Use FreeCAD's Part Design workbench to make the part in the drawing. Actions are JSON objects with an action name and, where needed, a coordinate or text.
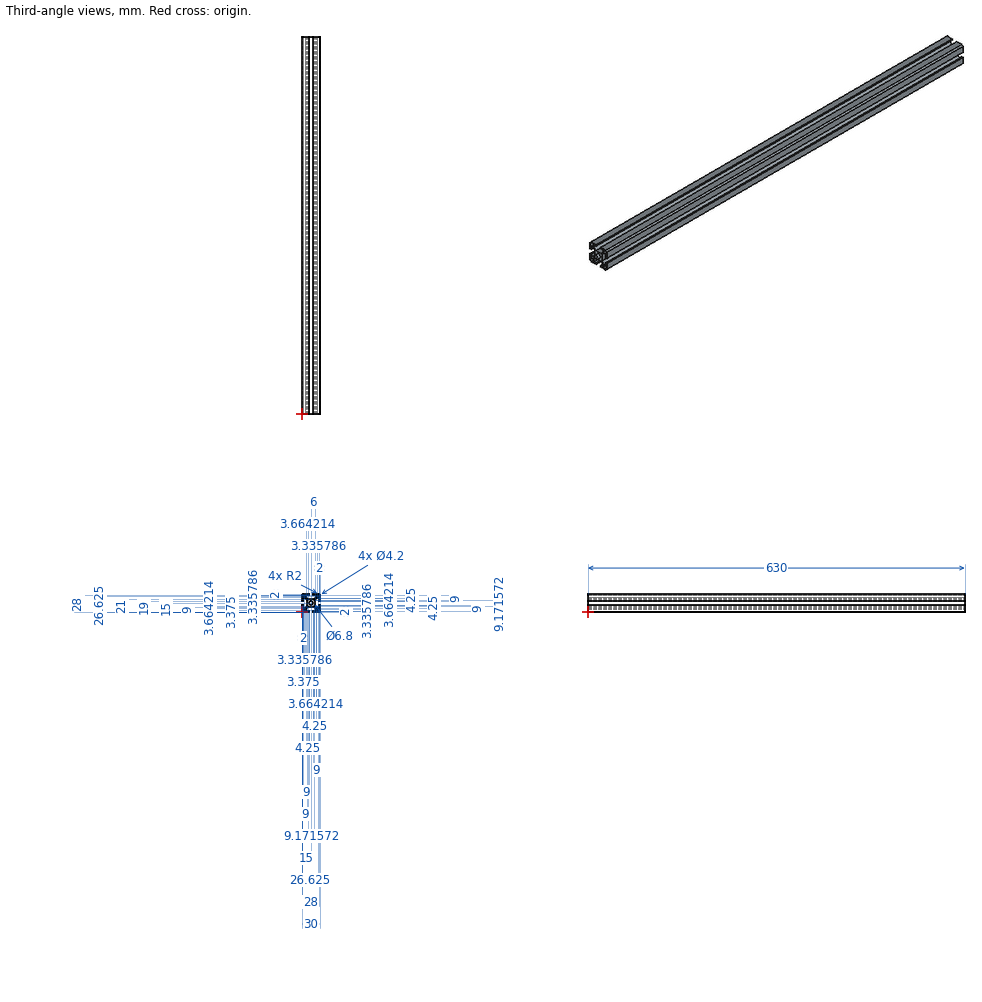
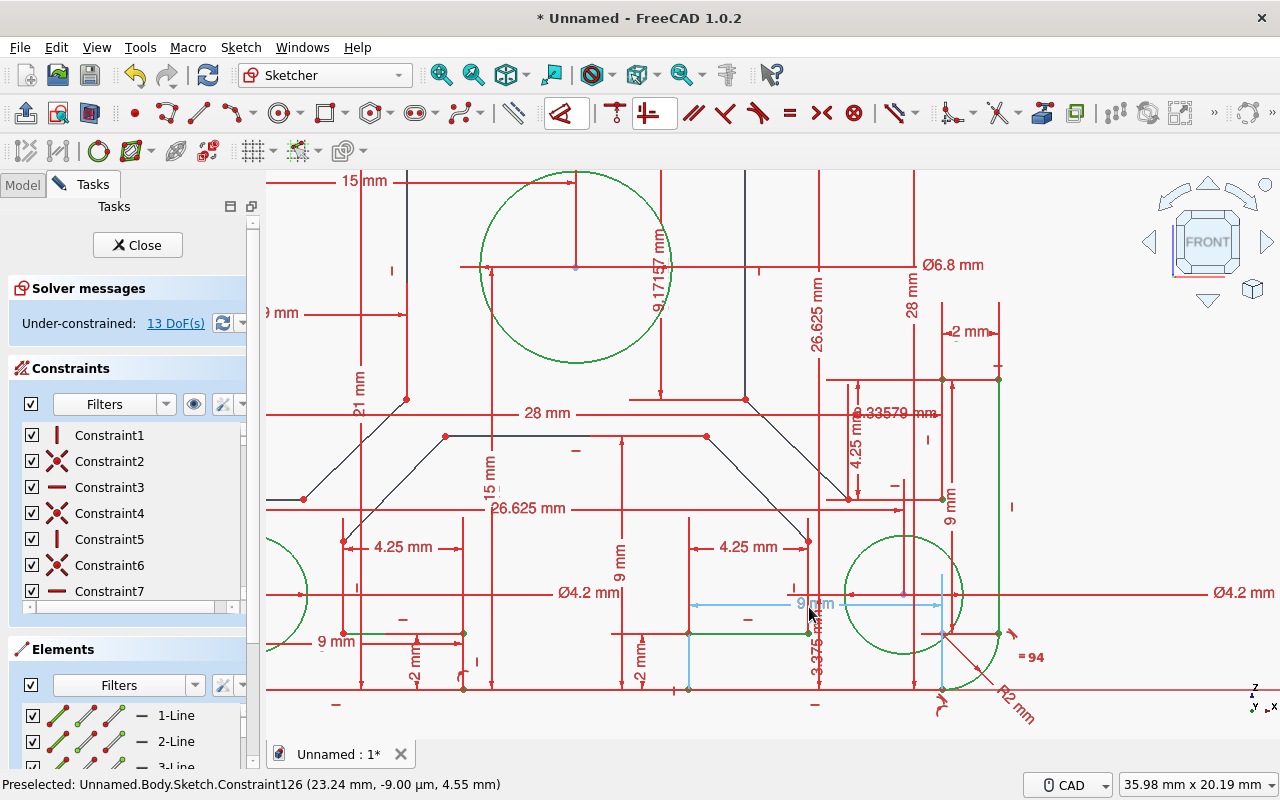
{"action": "left_click", "coordinate": [808, 569]}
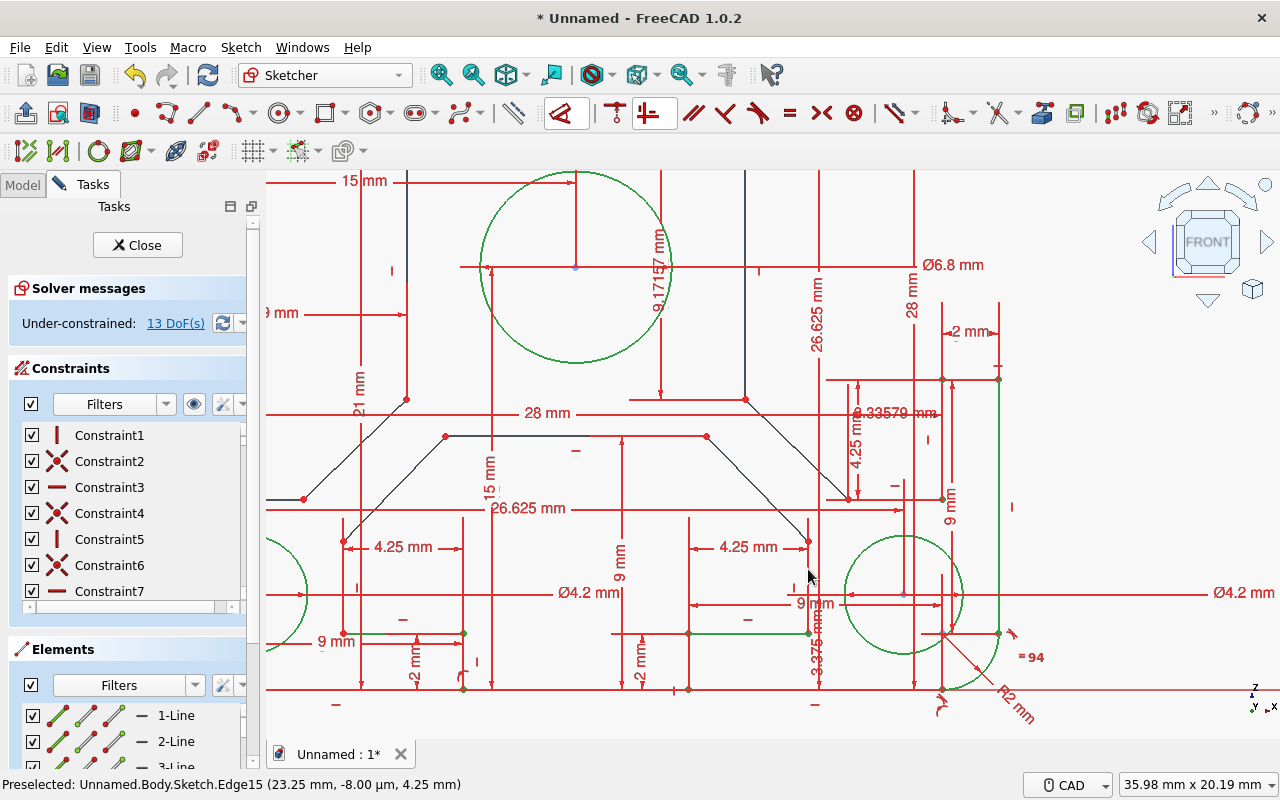
{"action": "key", "text": "i"}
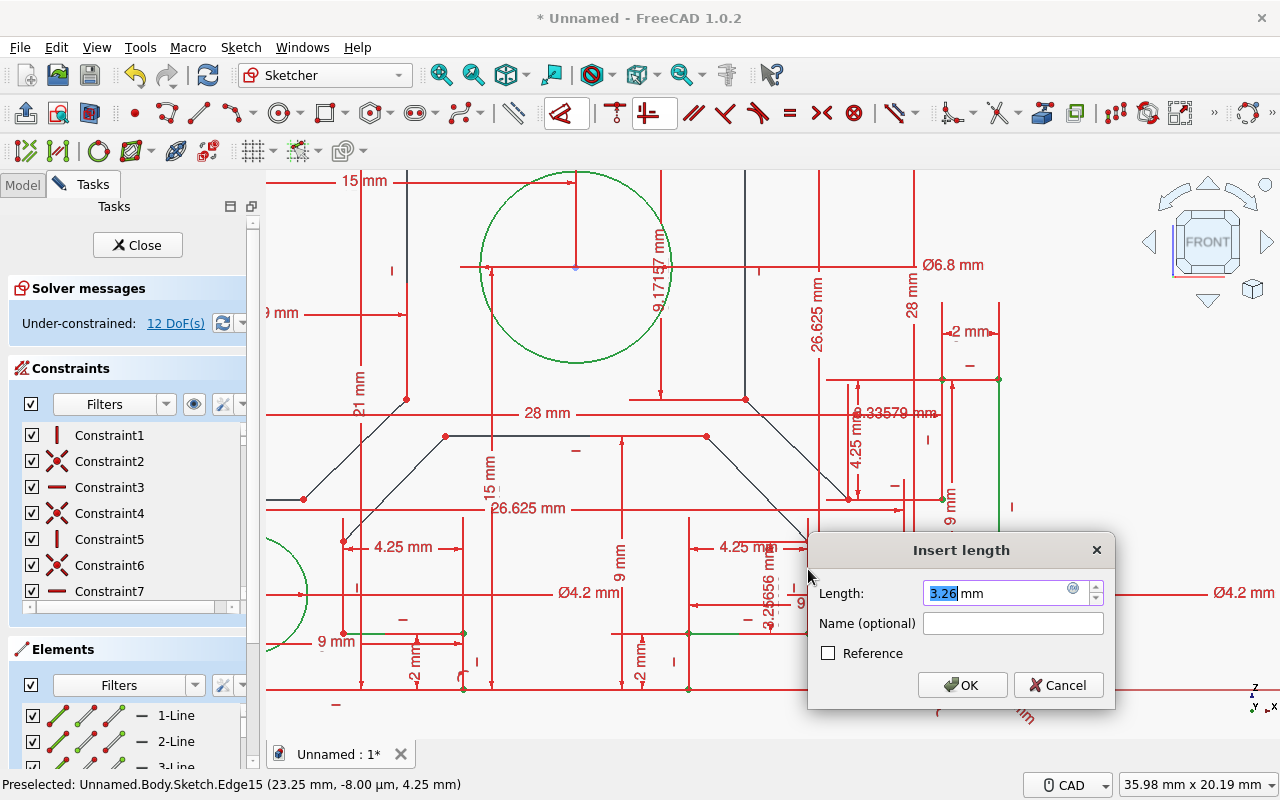
{"action": "type", "text": "3.335786"}
{"action": "key", "text": "Return"}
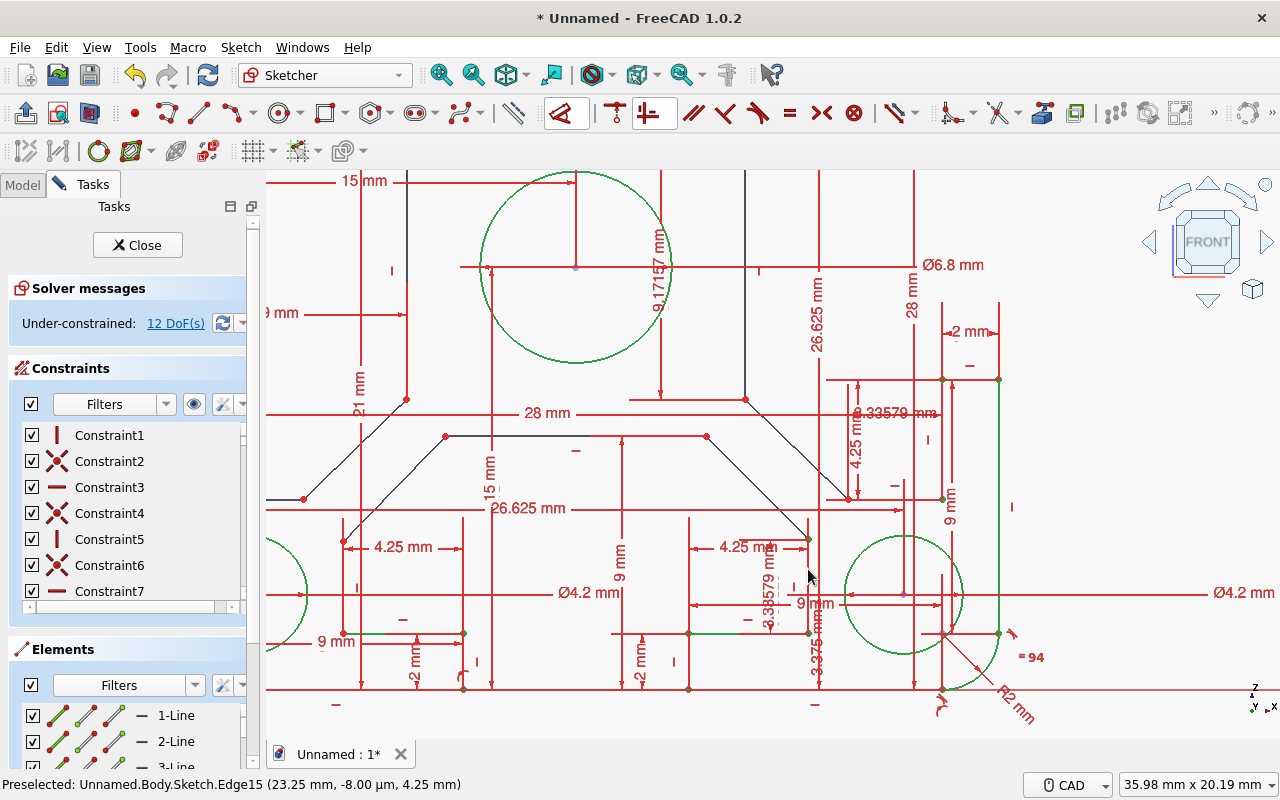
{"action": "left_click", "coordinate": [628, 436]}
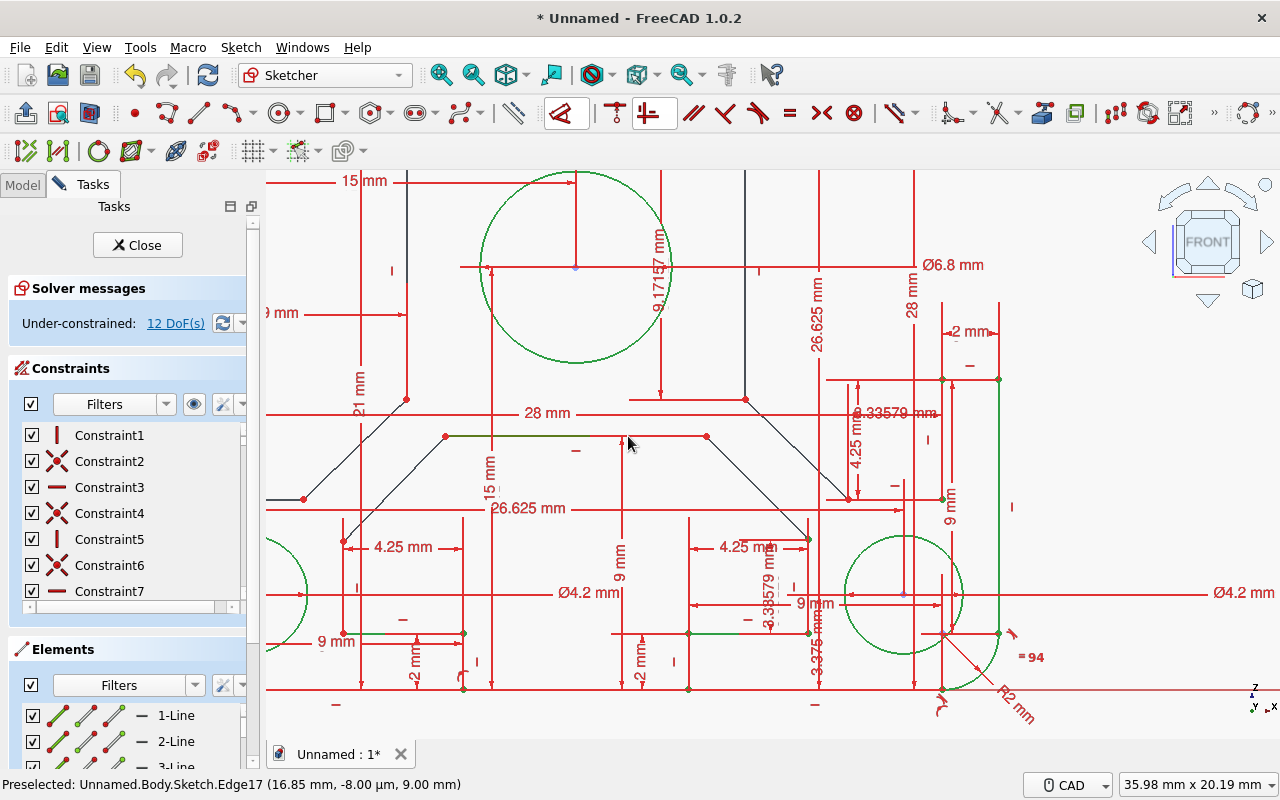
{"action": "left_click", "coordinate": [584, 114]}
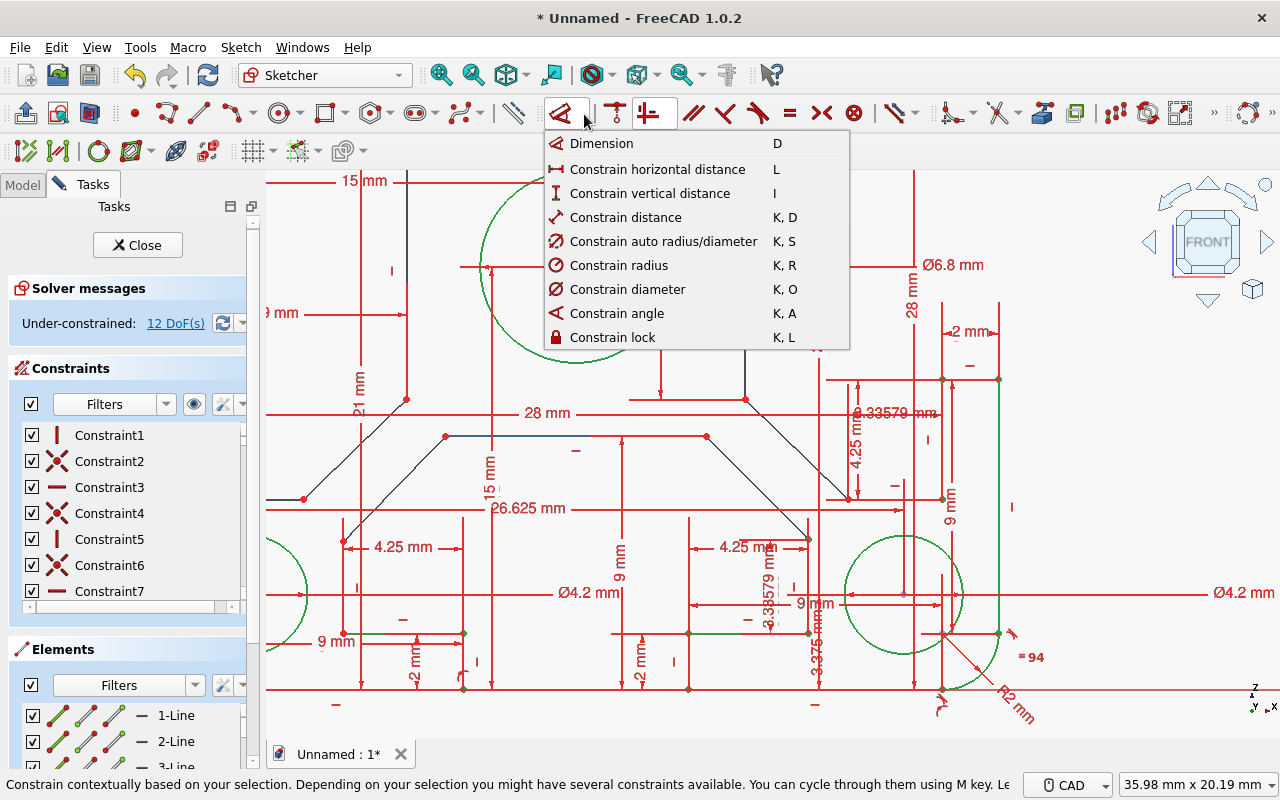
{"action": "left_click", "coordinate": [697, 169]}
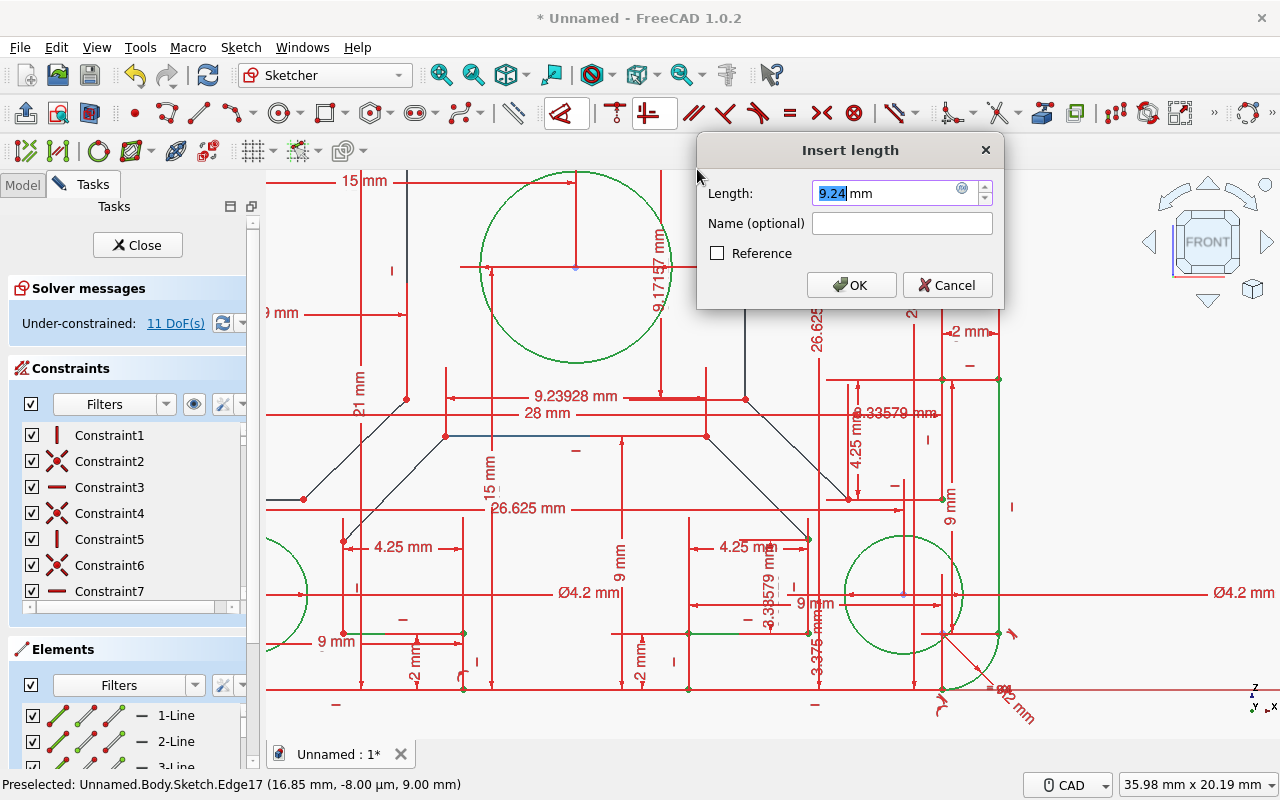
{"action": "type", "text": "9.171572"}
{"action": "key", "text": "Return"}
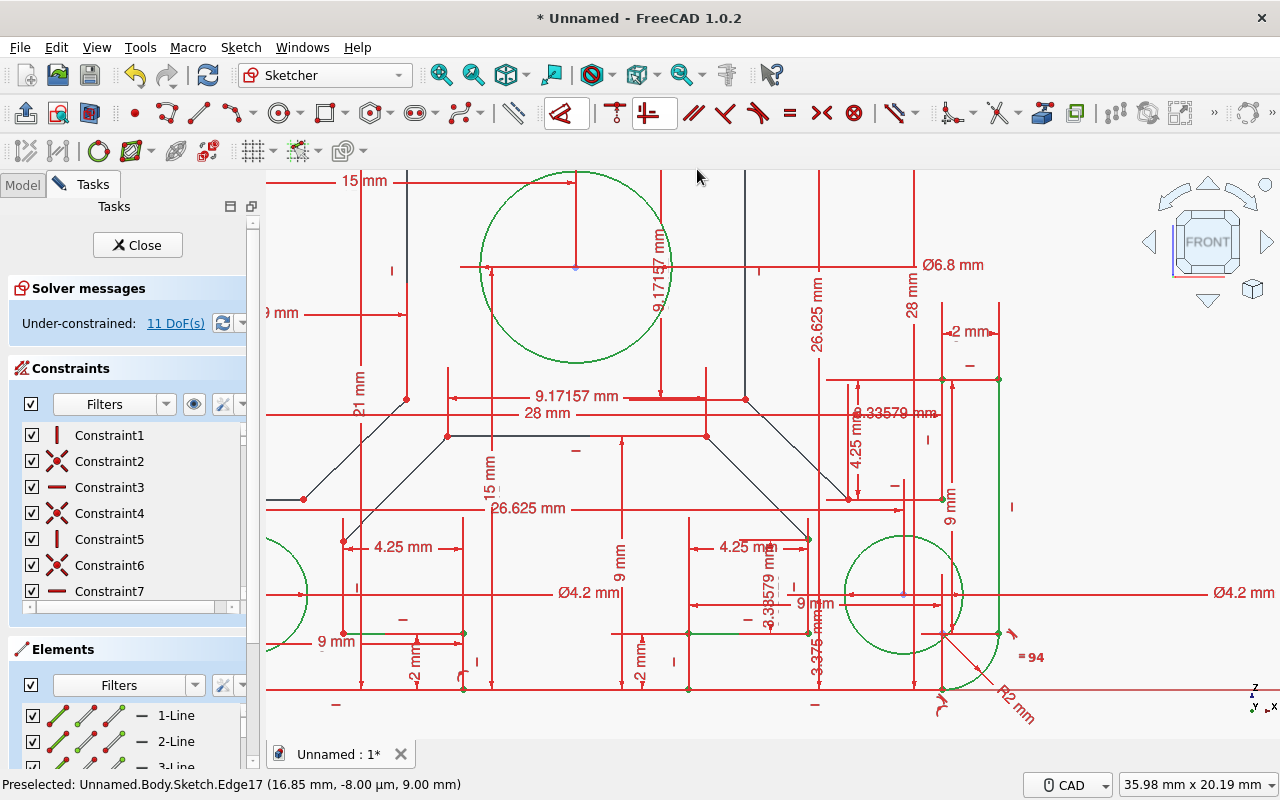
{"action": "left_click", "coordinate": [343, 569]}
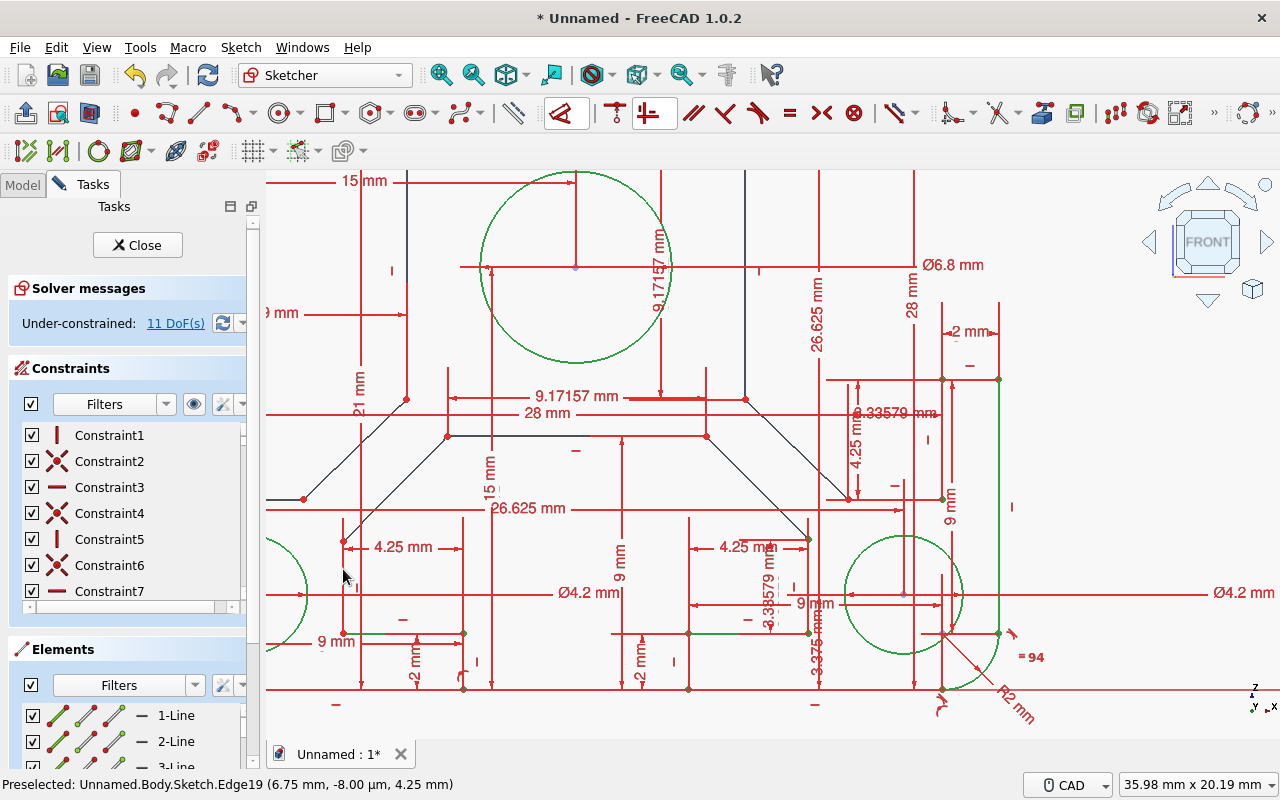
{"action": "key", "text": "i"}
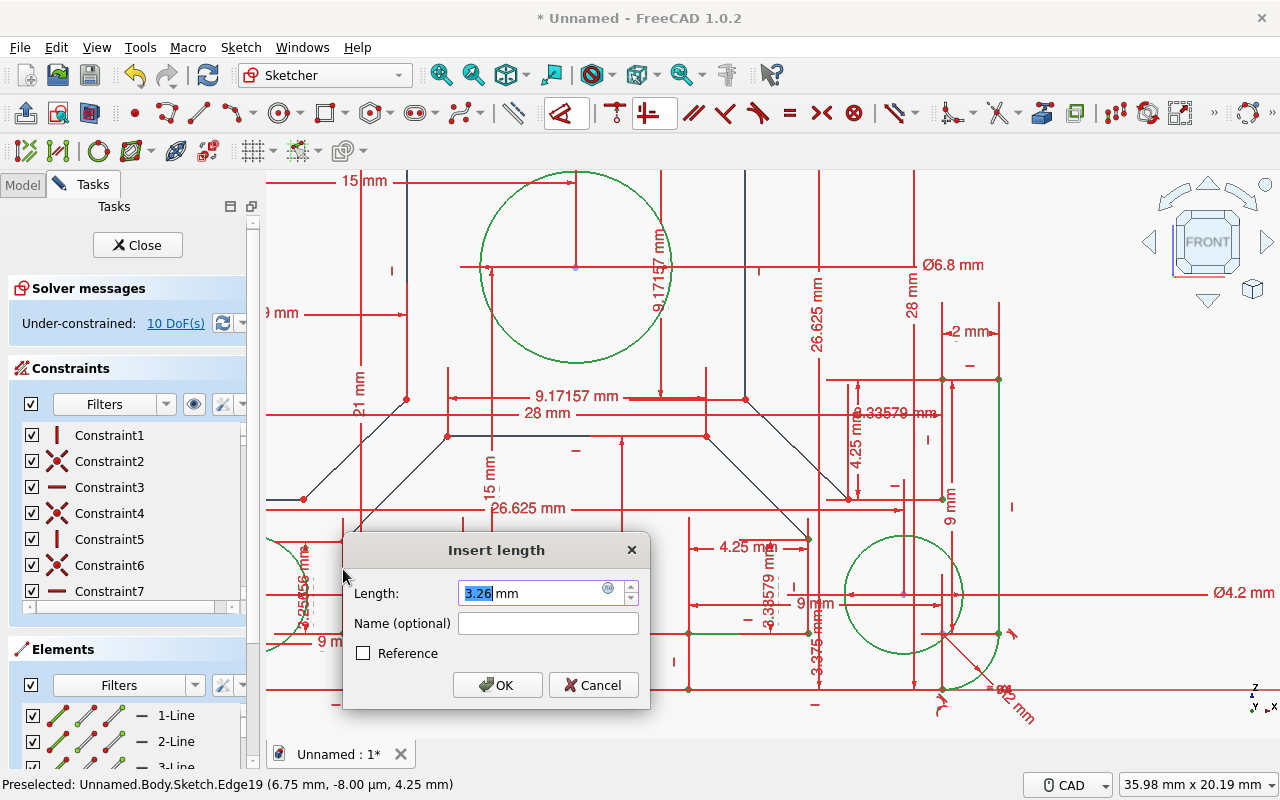
{"action": "type", "text": "3.335786"}
{"action": "key", "text": "Return"}